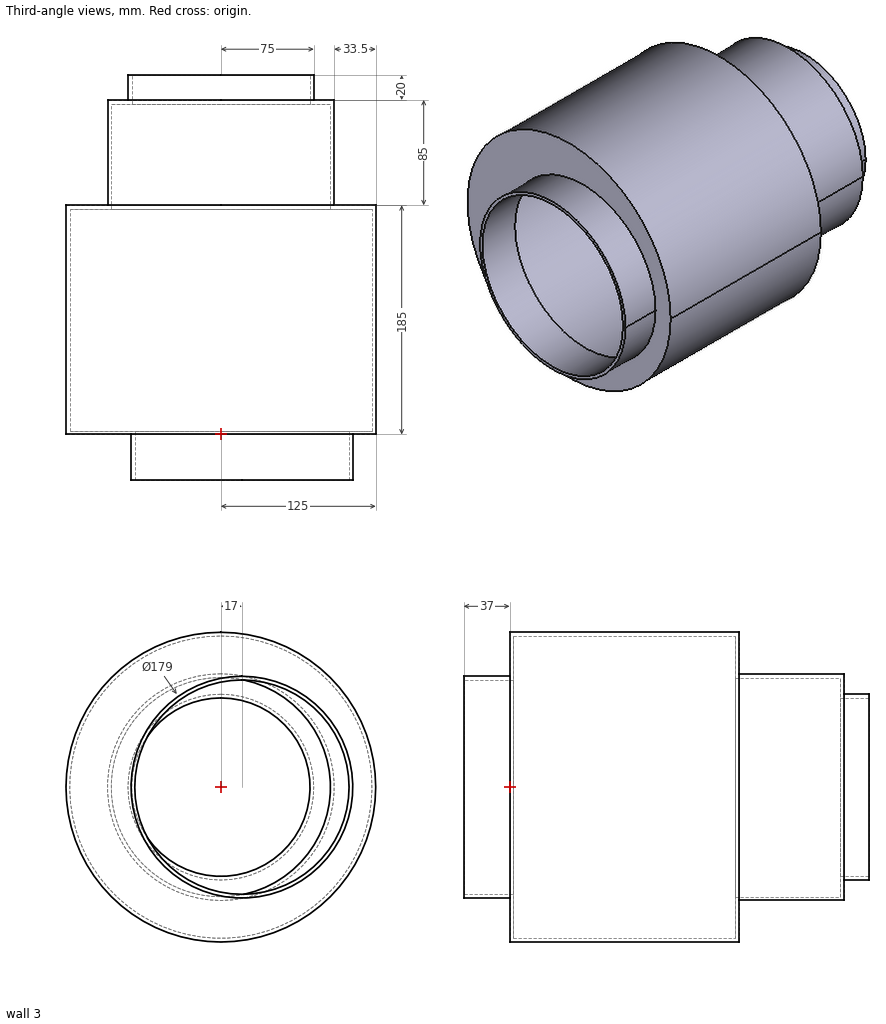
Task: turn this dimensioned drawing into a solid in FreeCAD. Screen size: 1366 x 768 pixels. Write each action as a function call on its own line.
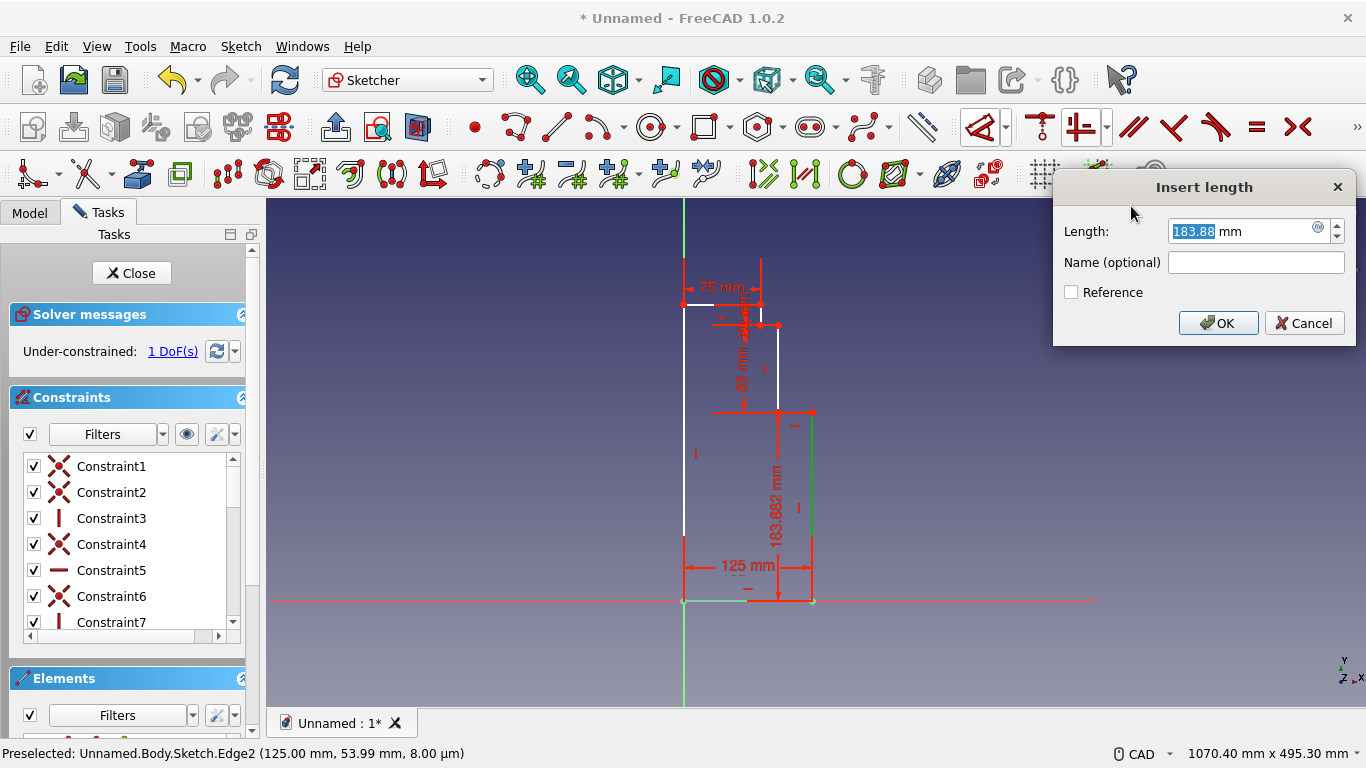
text(185)
key(Return)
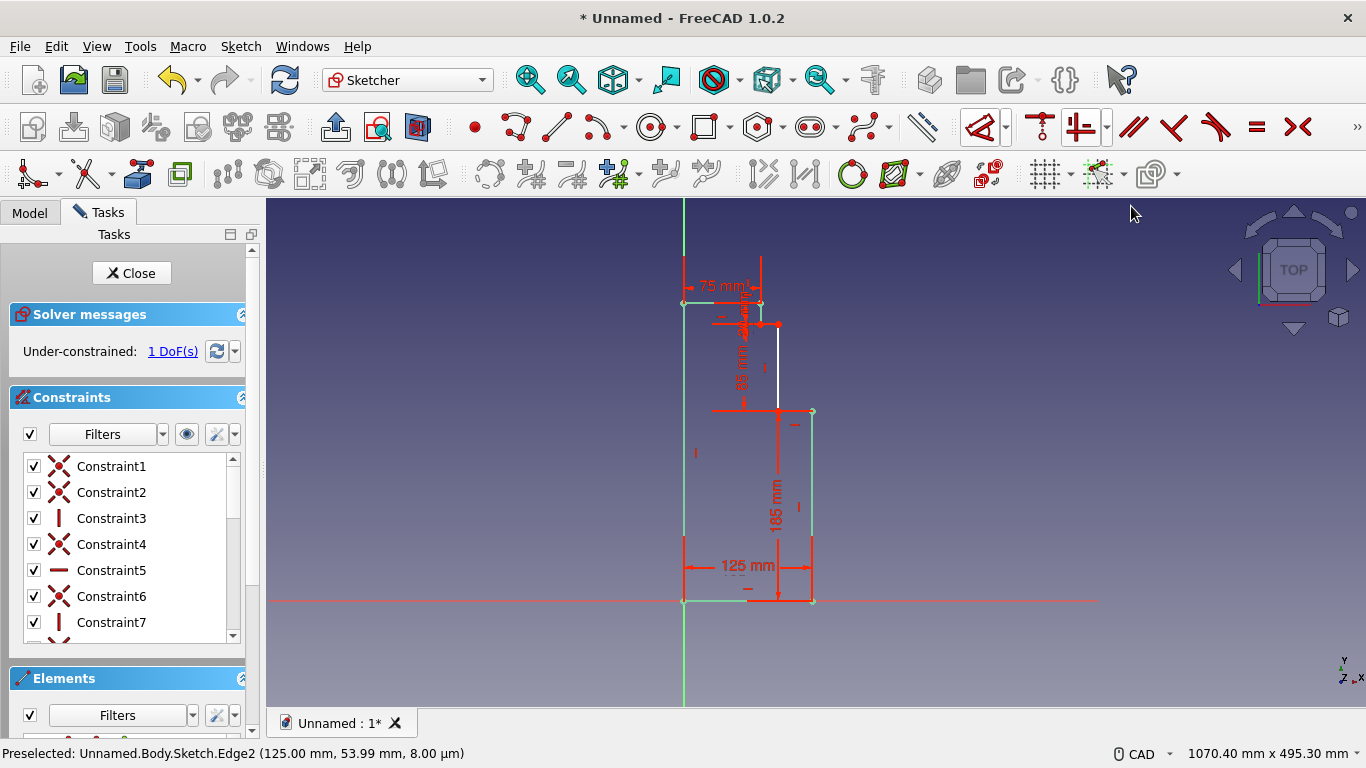
scroll(802, 411, up, 2)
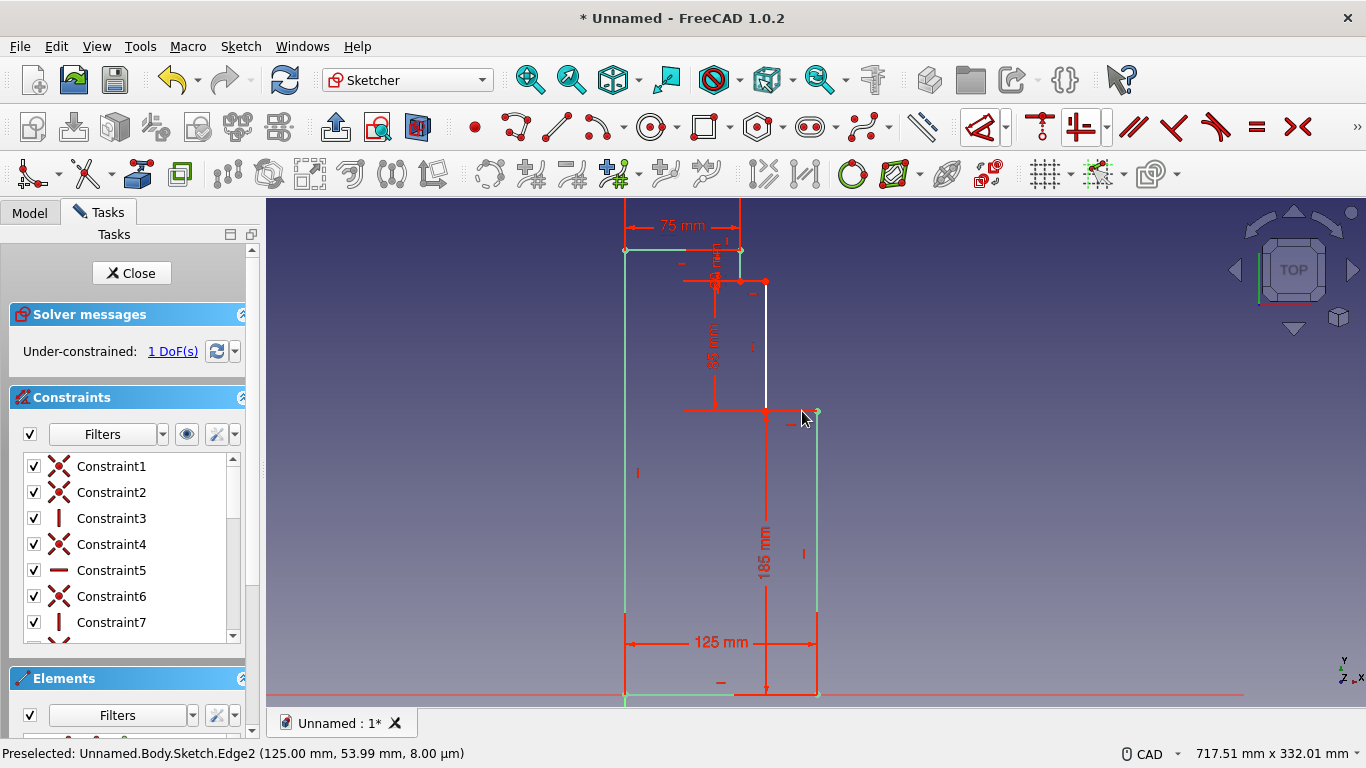
click(802, 411)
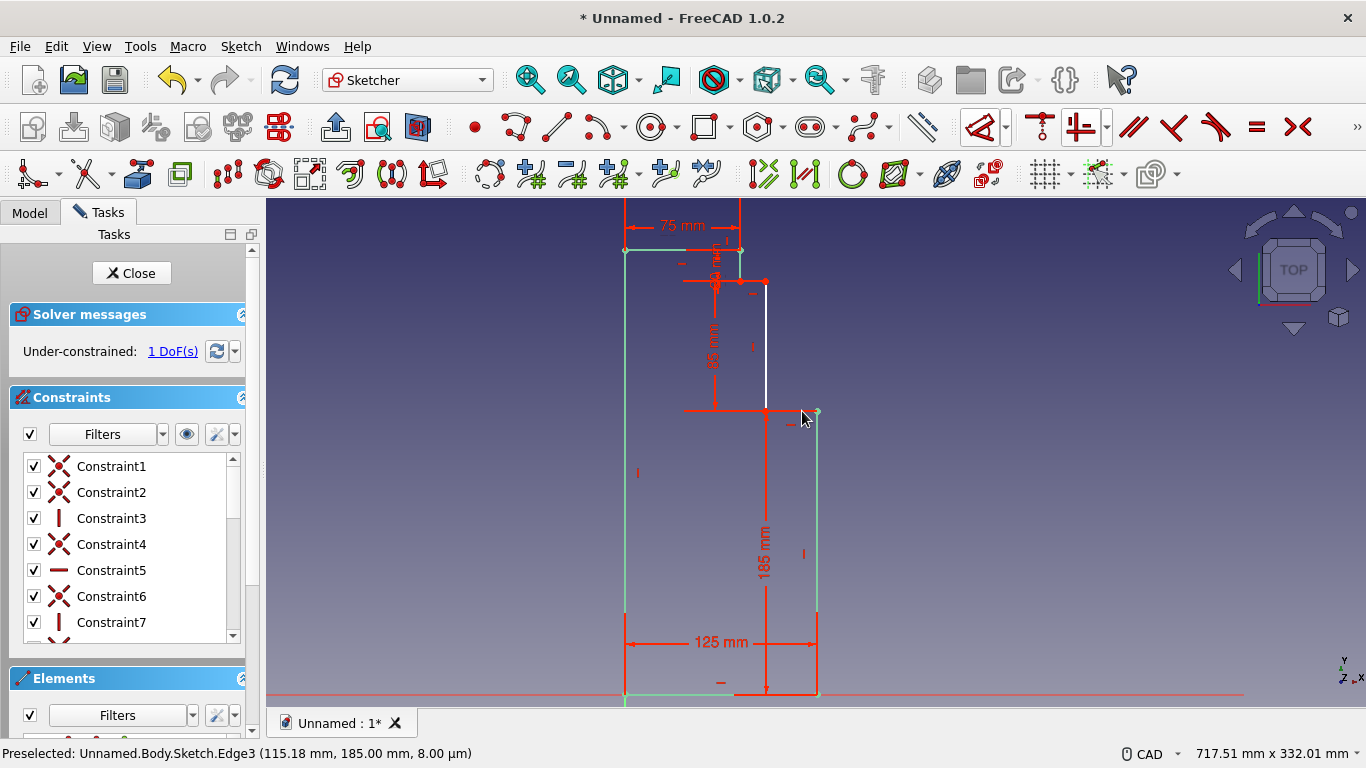
click(1006, 128)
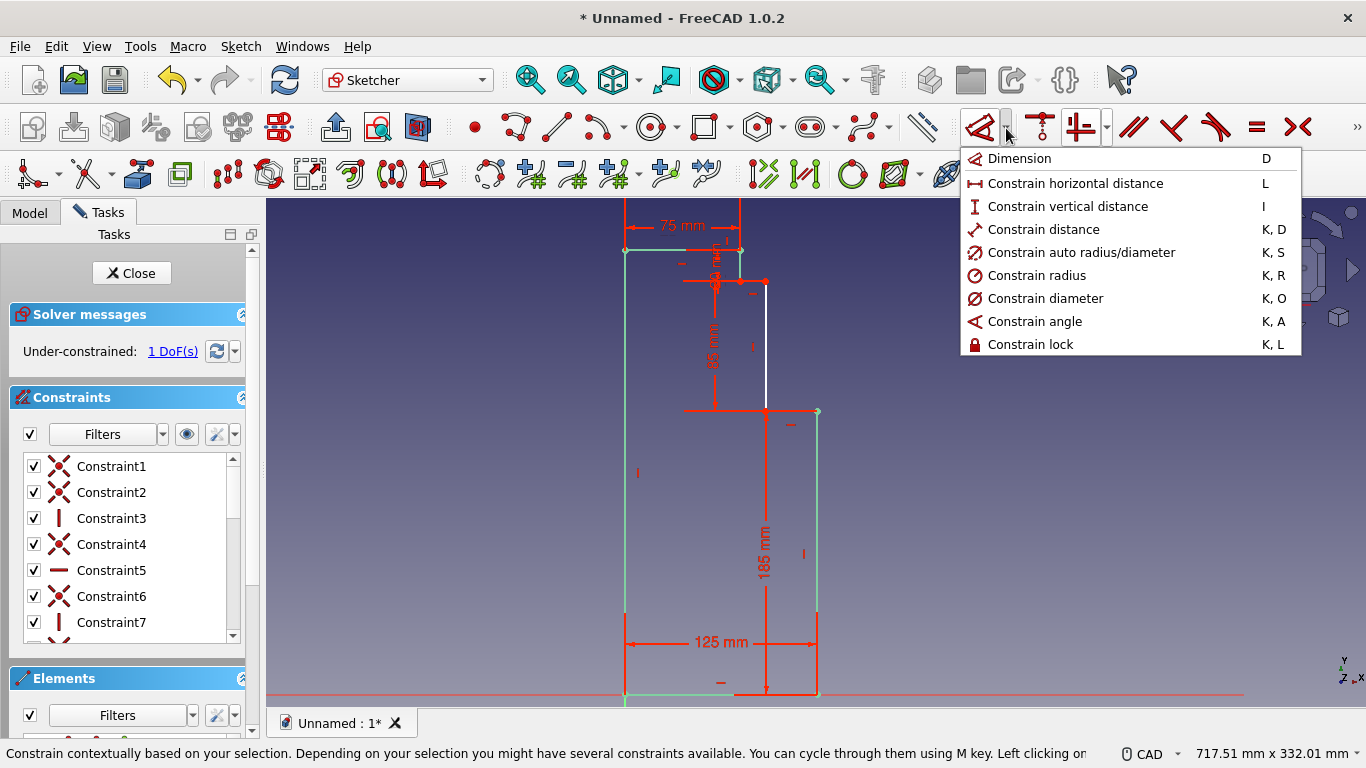
click(1131, 184)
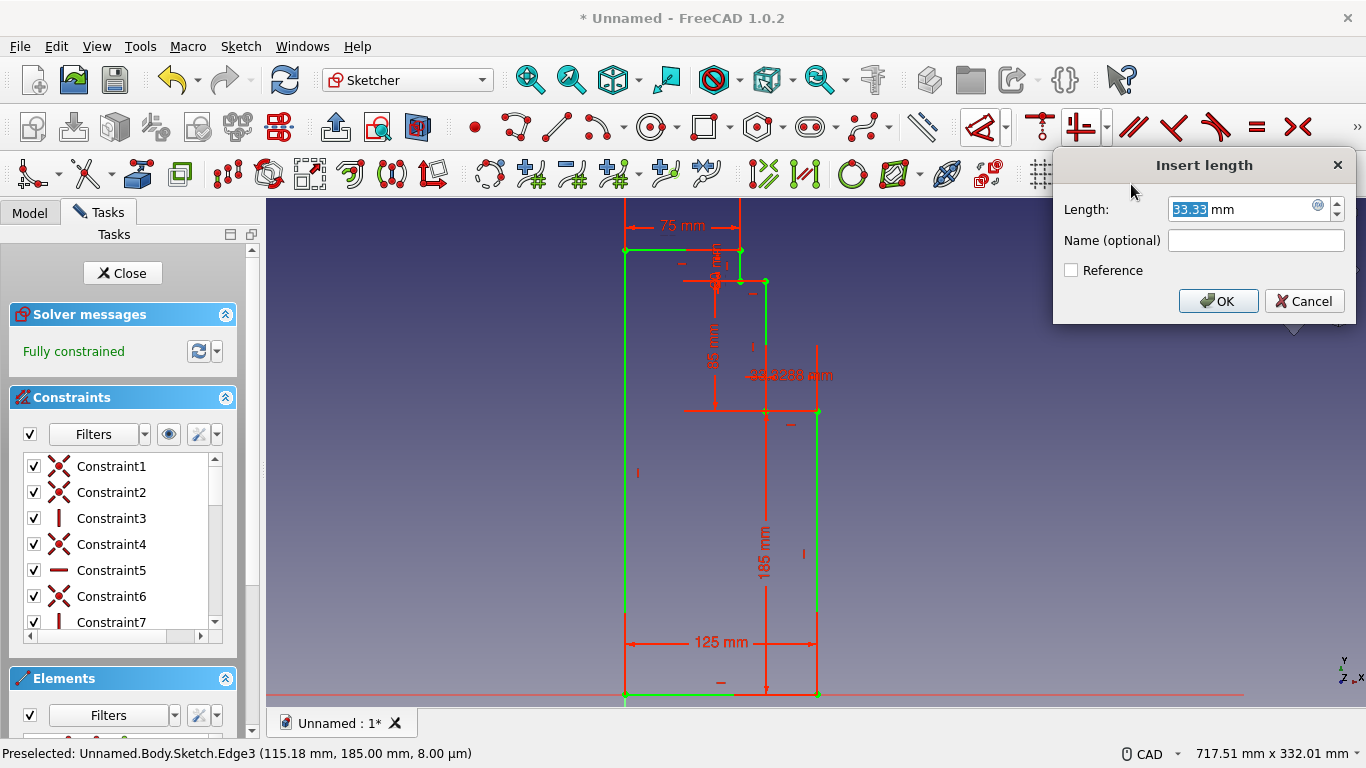
text(33.5)
key(Return)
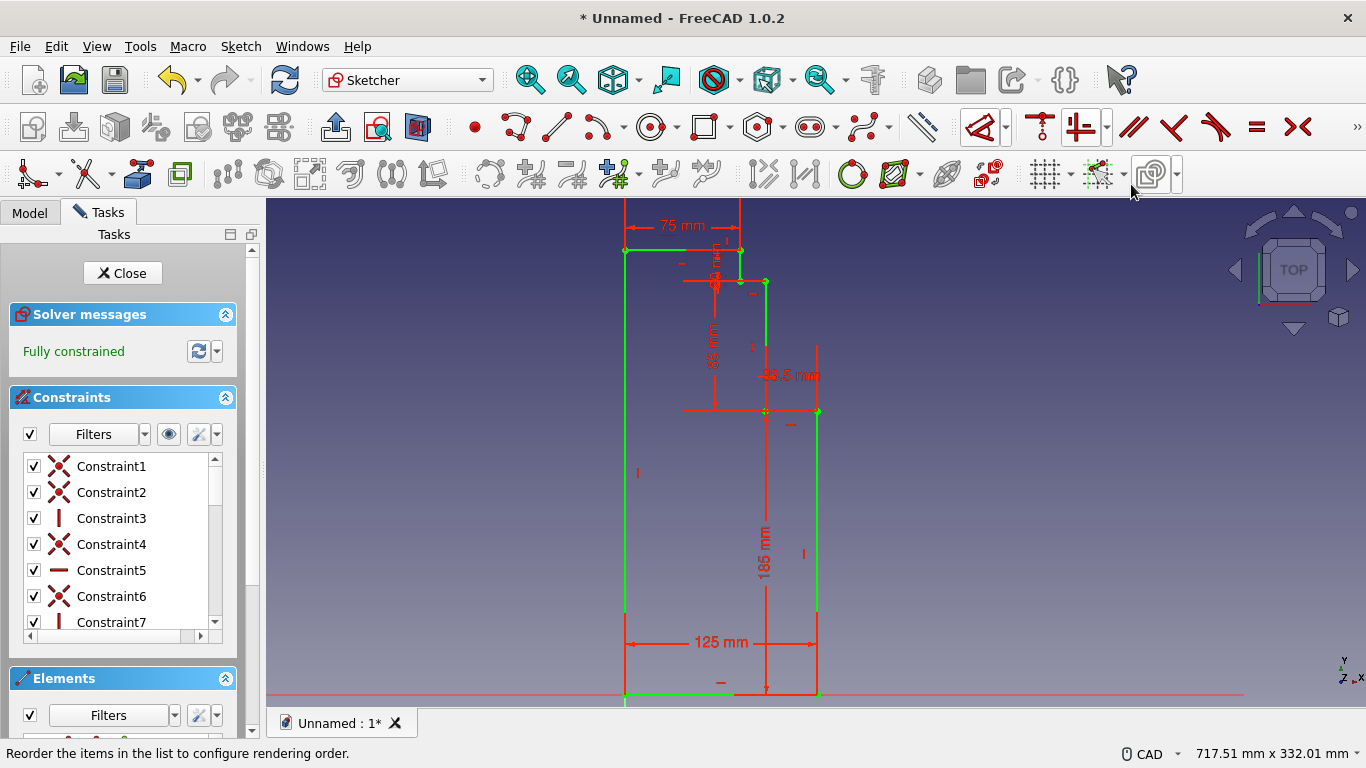
click(123, 273)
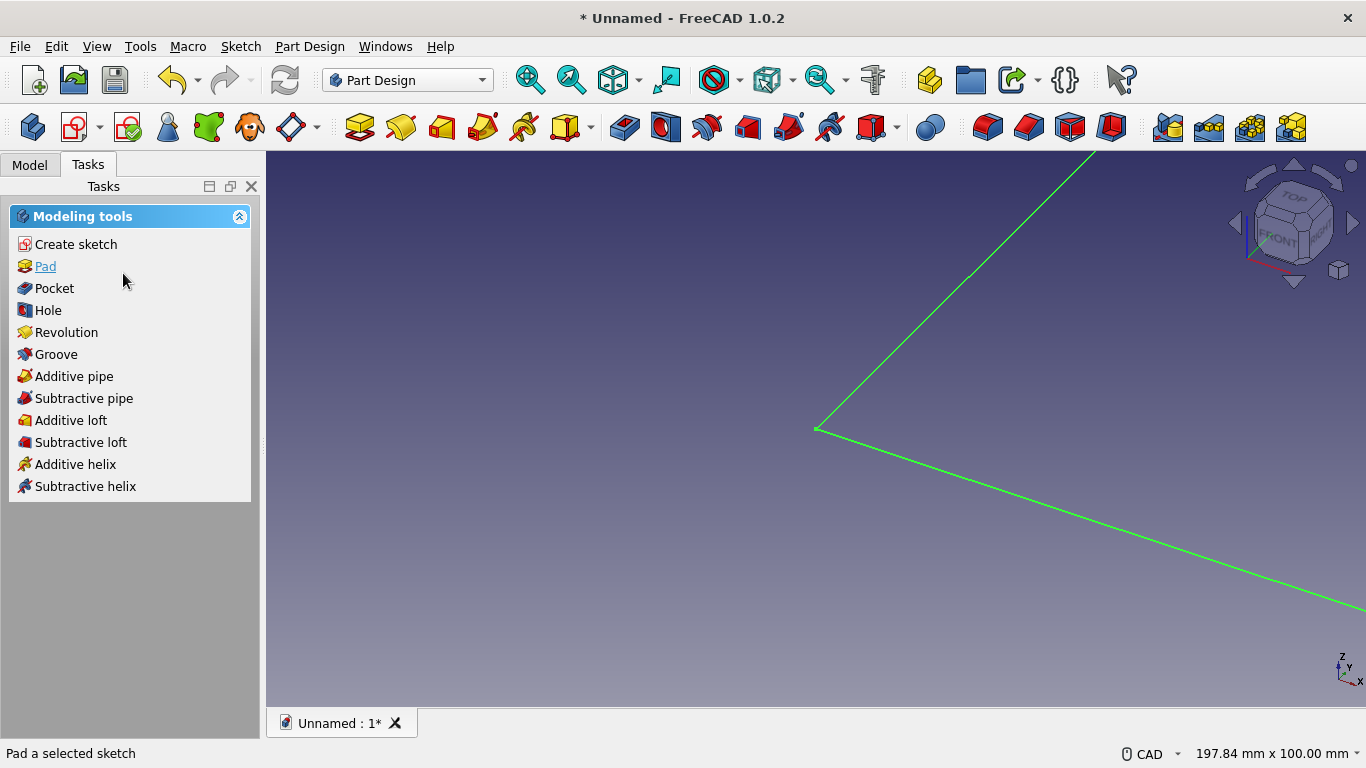
click(401, 128)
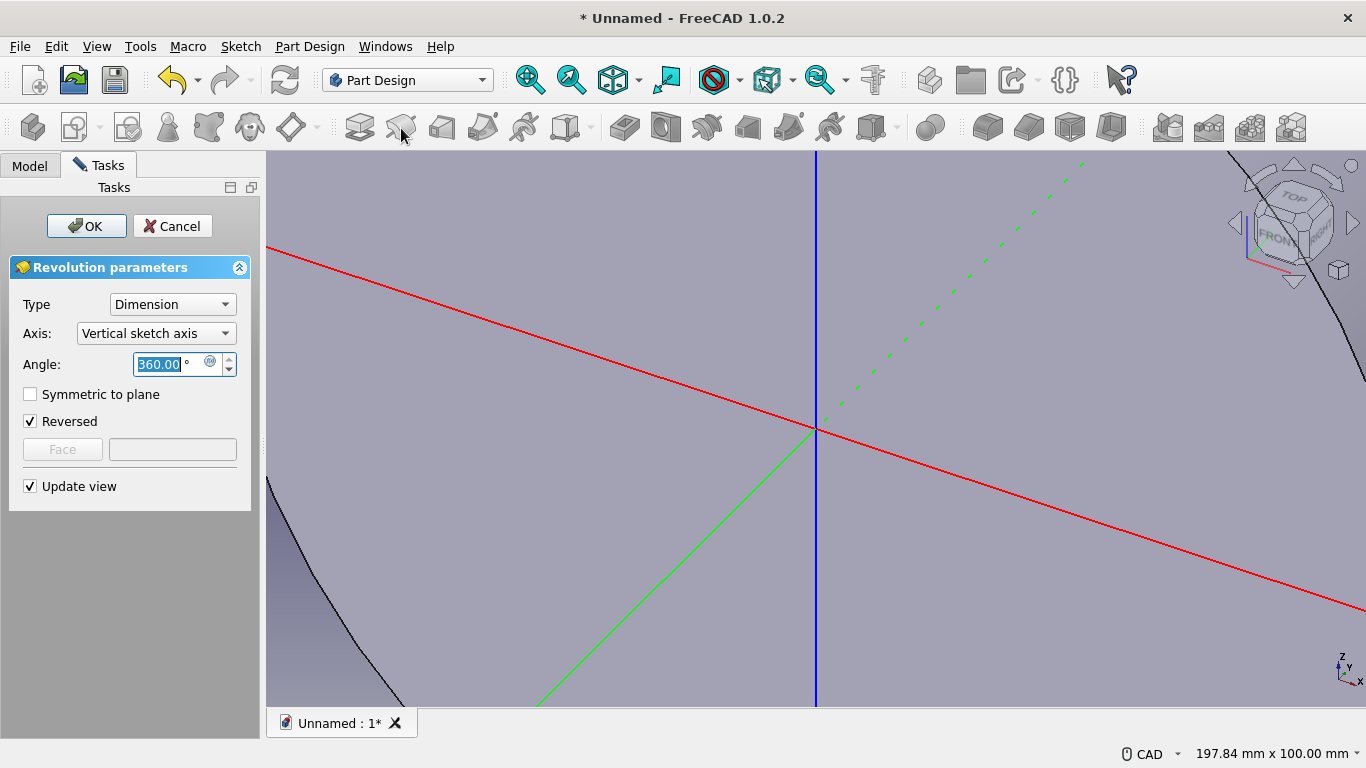
click(87, 226)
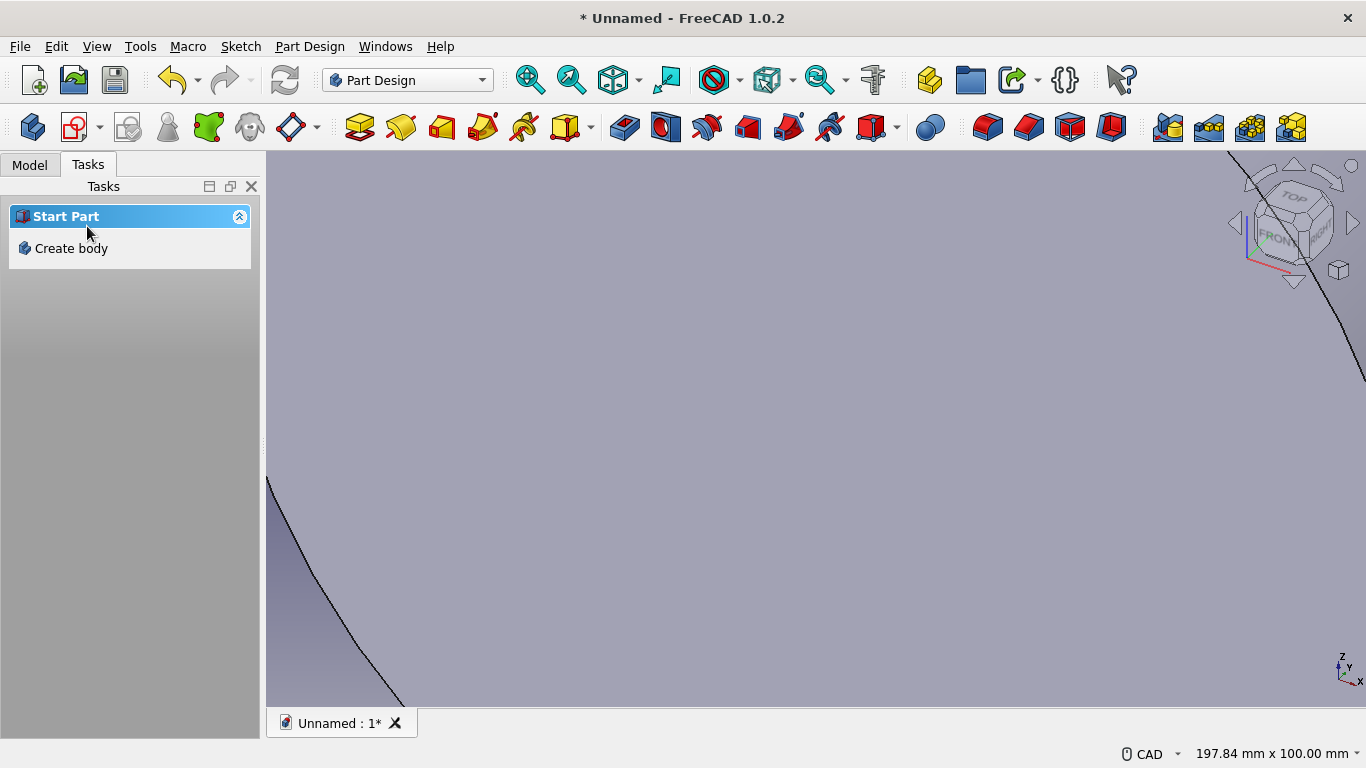
click(531, 80)